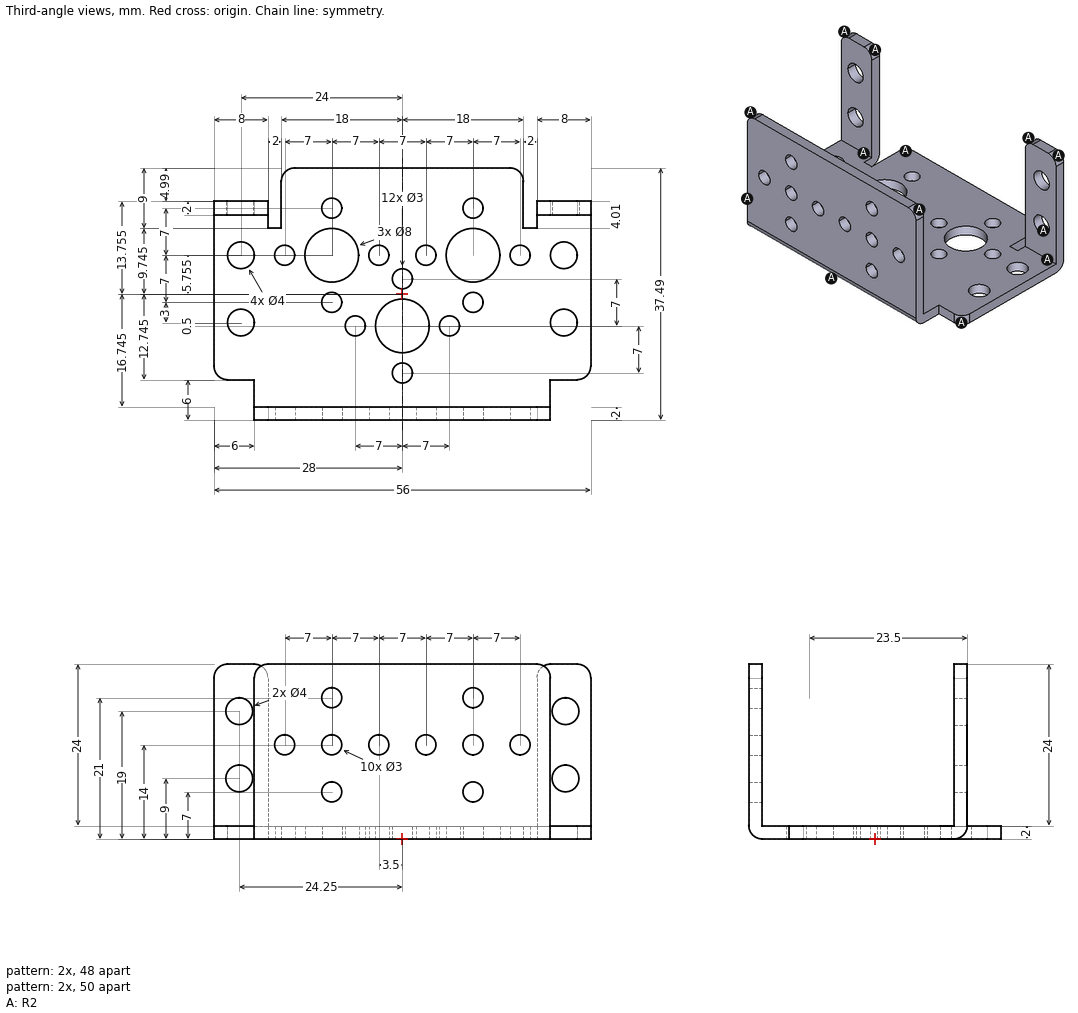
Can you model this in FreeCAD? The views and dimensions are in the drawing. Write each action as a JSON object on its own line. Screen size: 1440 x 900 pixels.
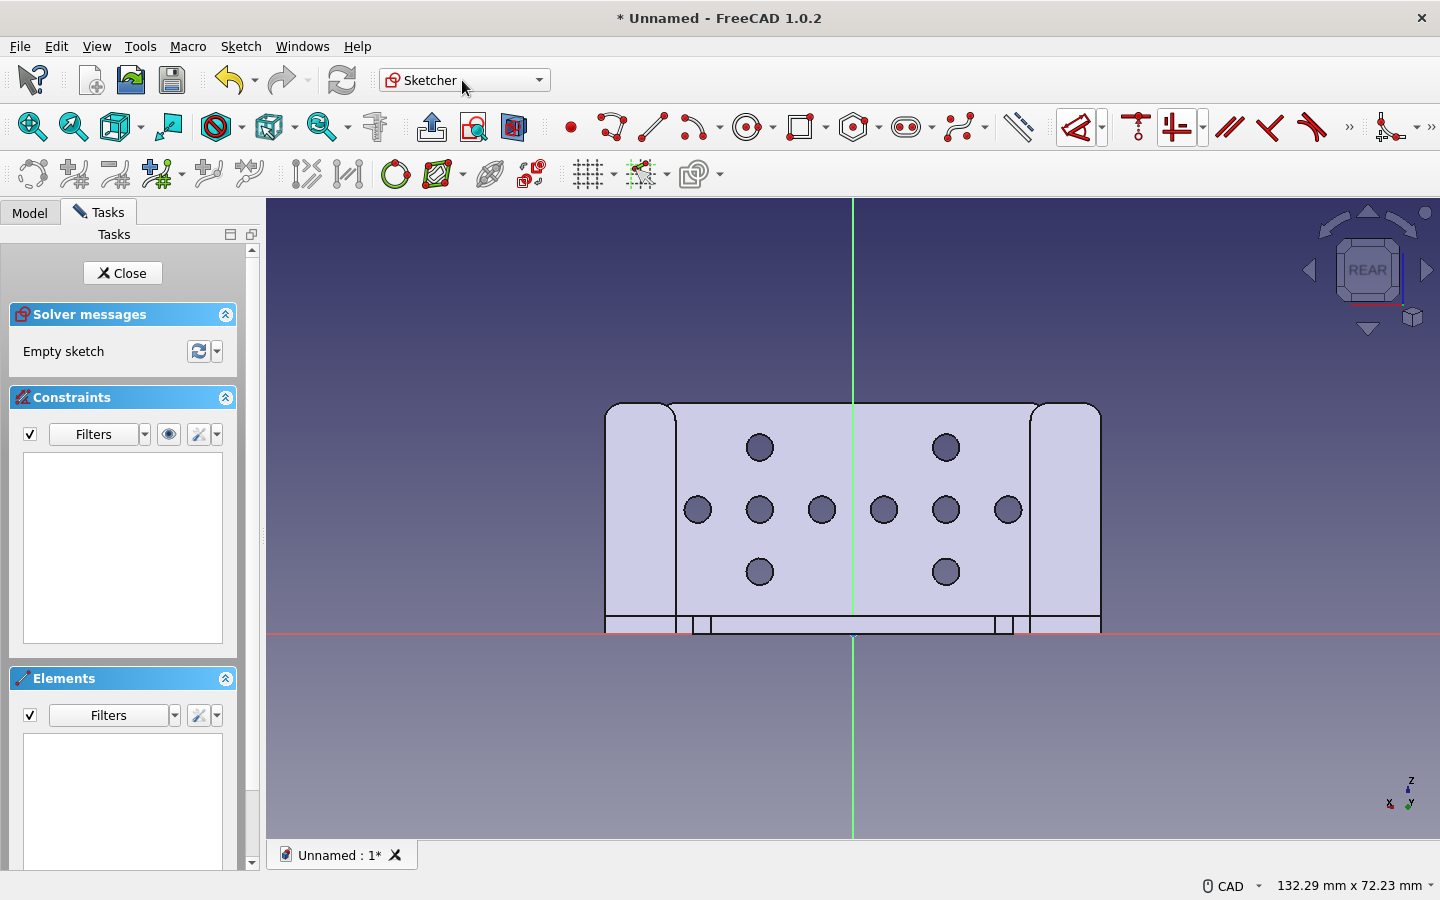
{"action": "key", "text": "q s"}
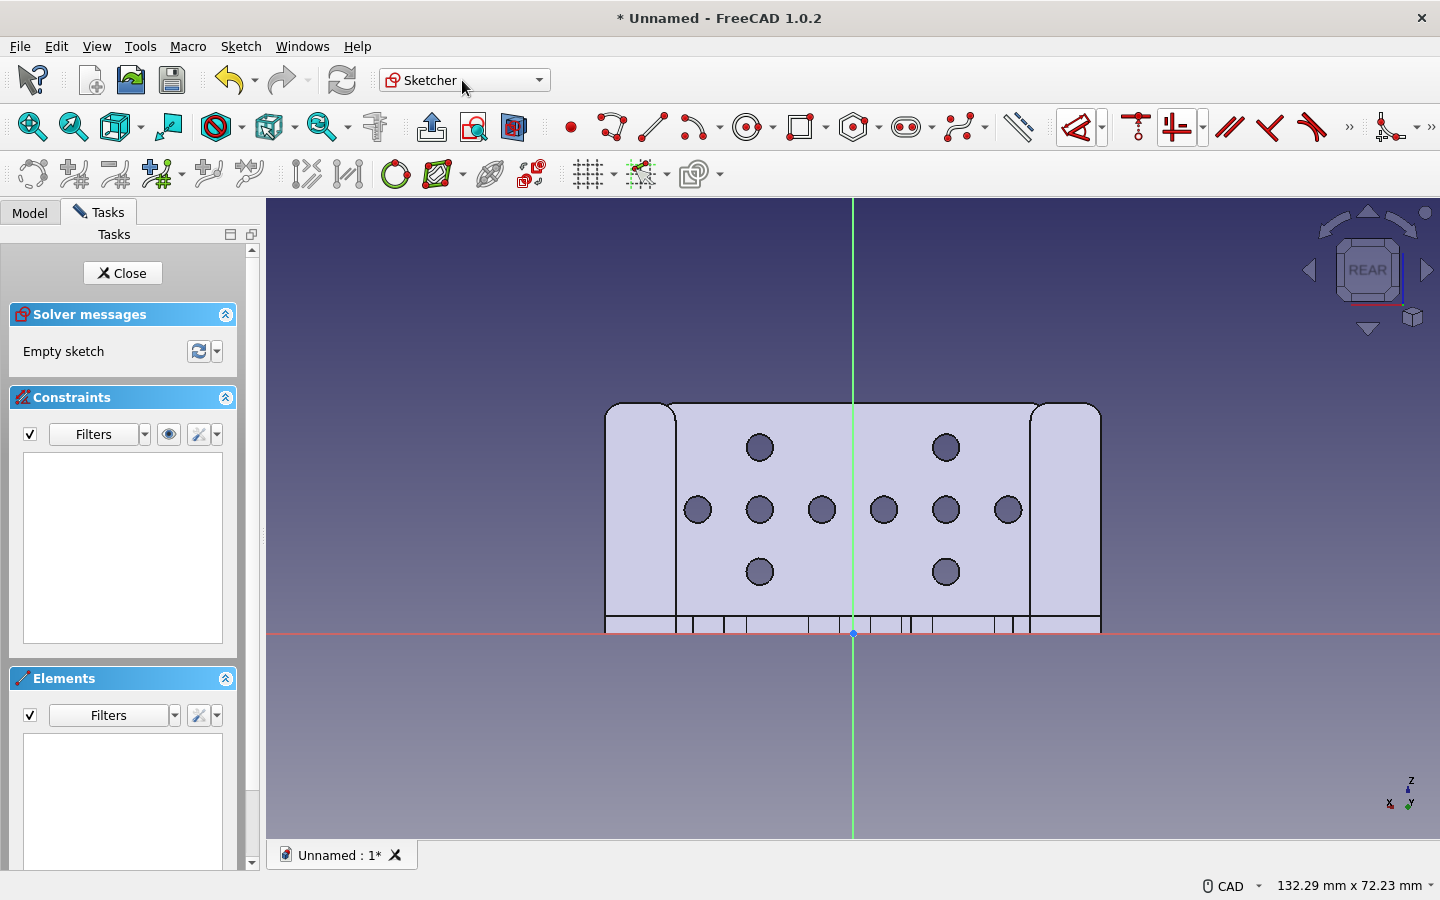
{"action": "scroll", "coordinate": [1120, 559], "scroll_direction": "up", "scroll_amount": 4}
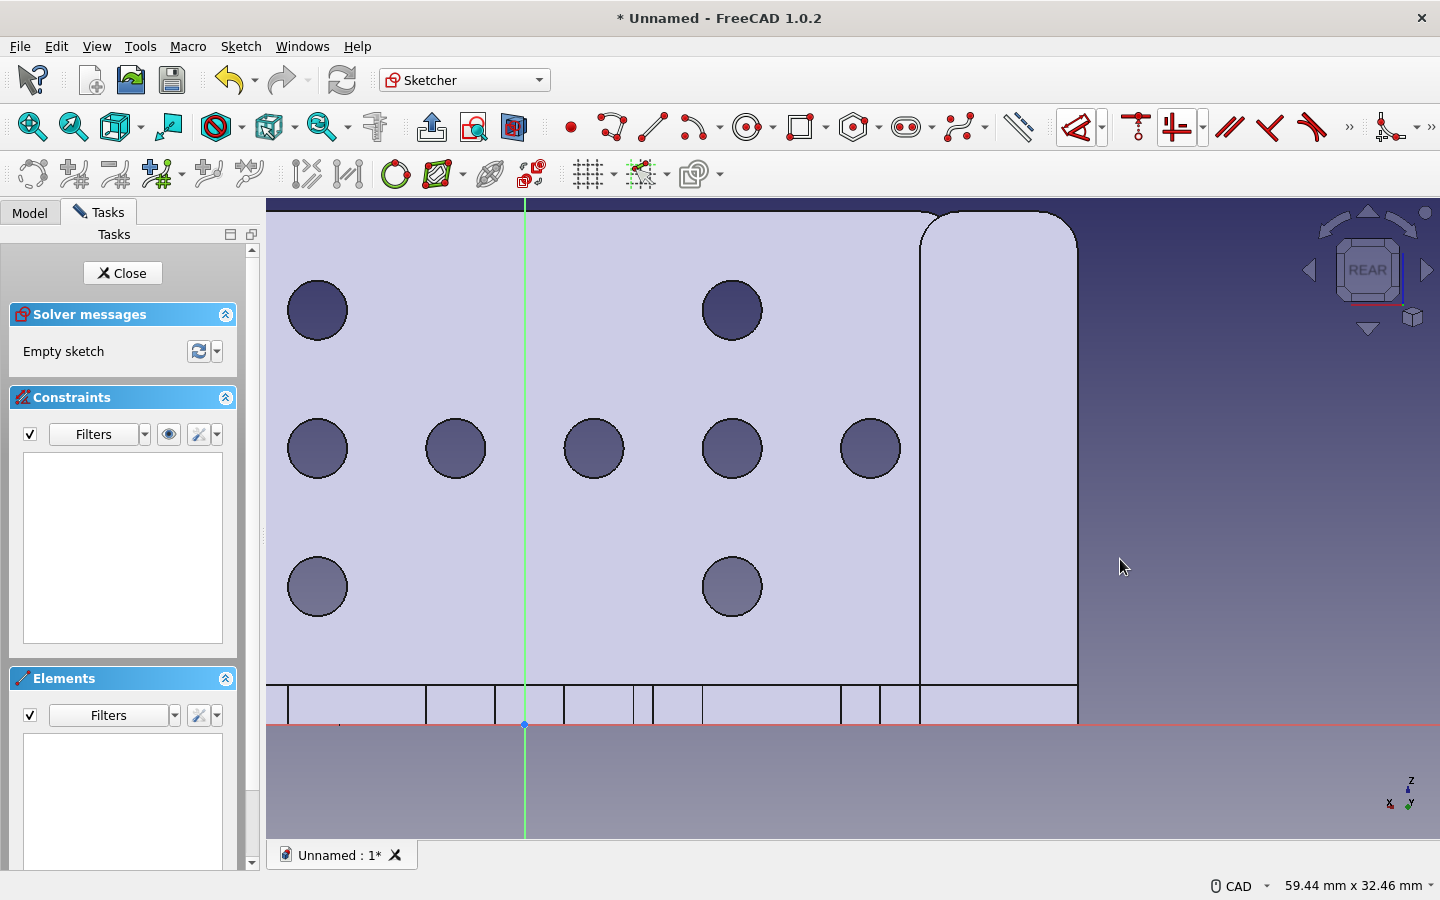
{"action": "left_click", "coordinate": [746, 128]}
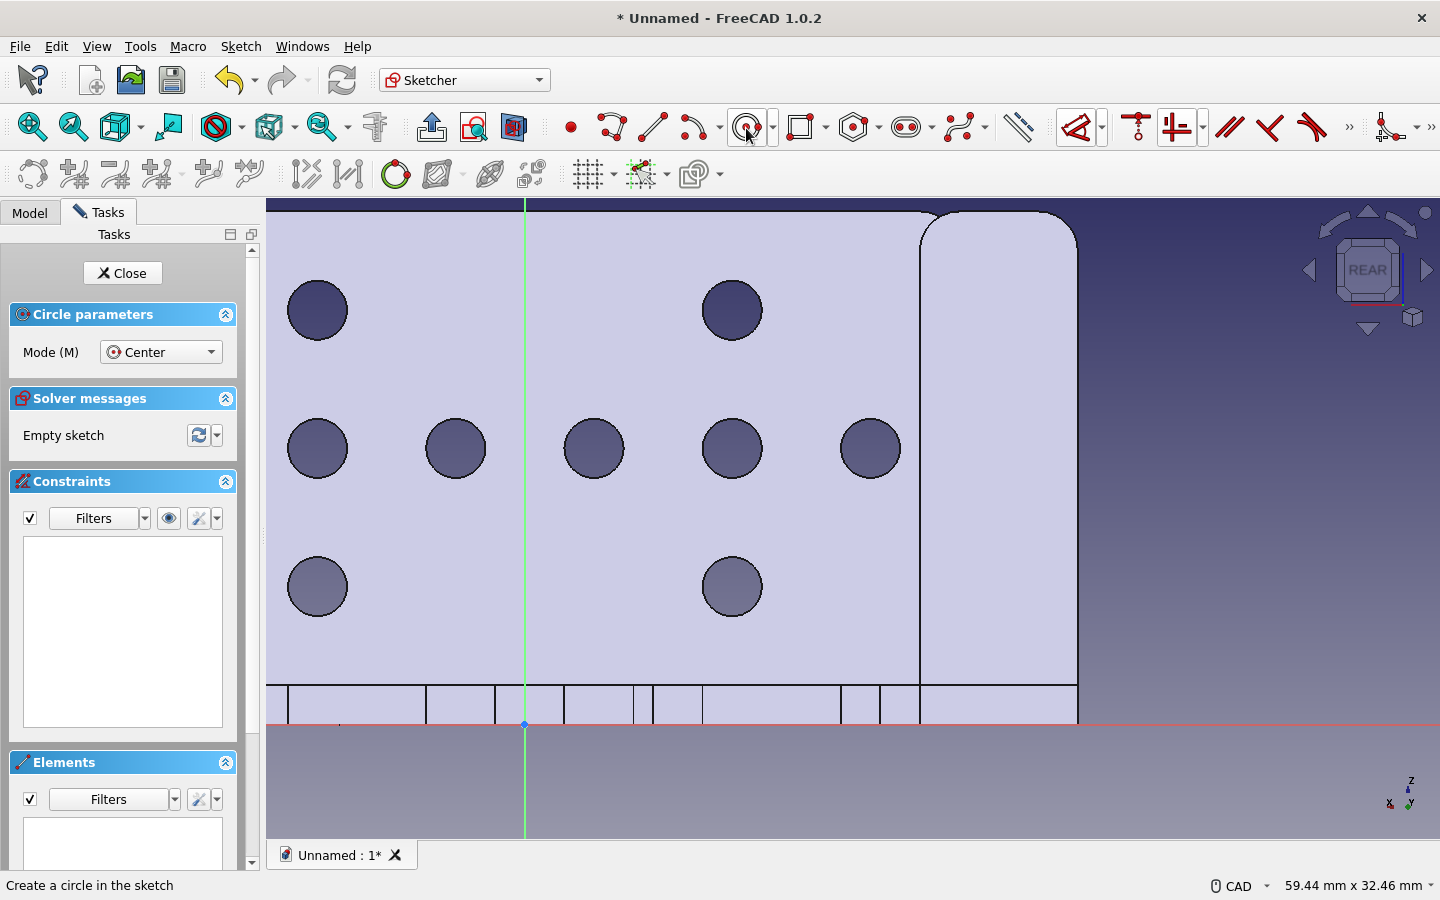
{"action": "left_click", "coordinate": [1004, 350]}
{"action": "mouse_move", "coordinate": [1032, 322]}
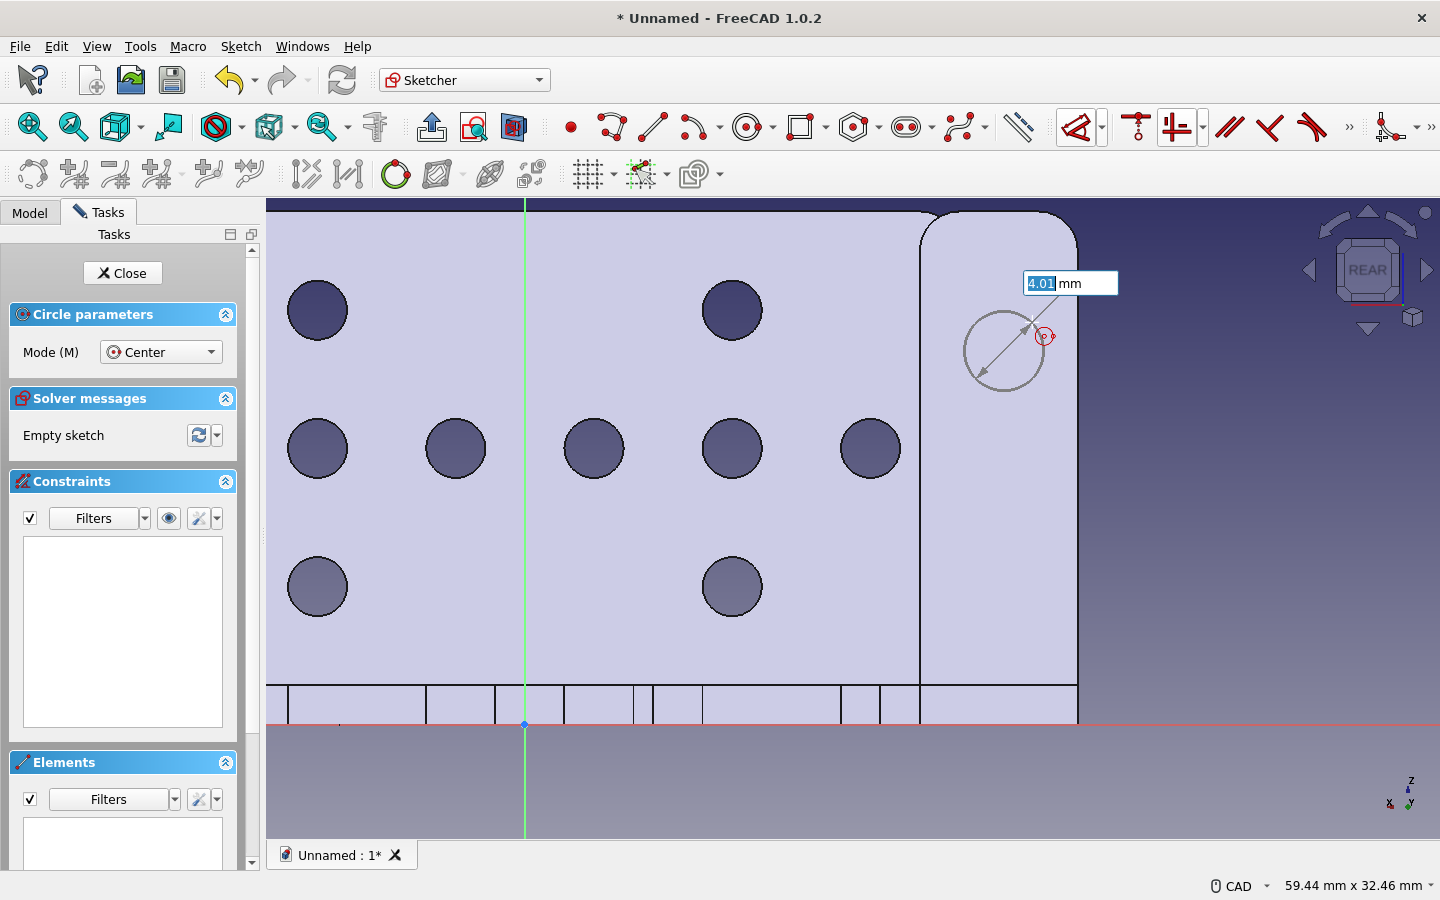
{"action": "type", "text": "4"}
{"action": "key", "text": "Return"}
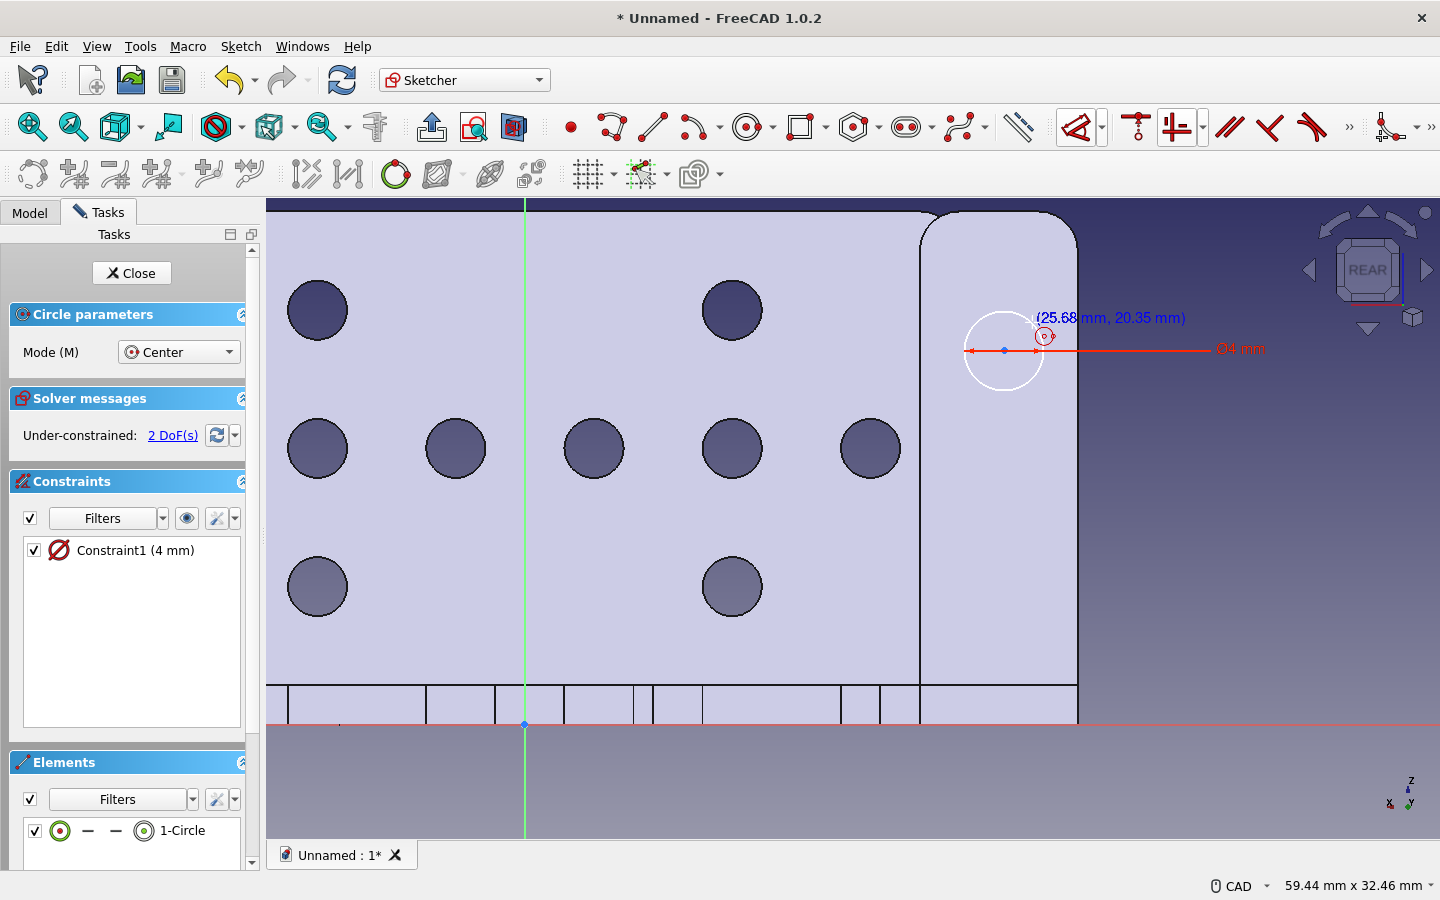
{"action": "left_click", "coordinate": [1004, 547]}
{"action": "mouse_move", "coordinate": [1032, 519]}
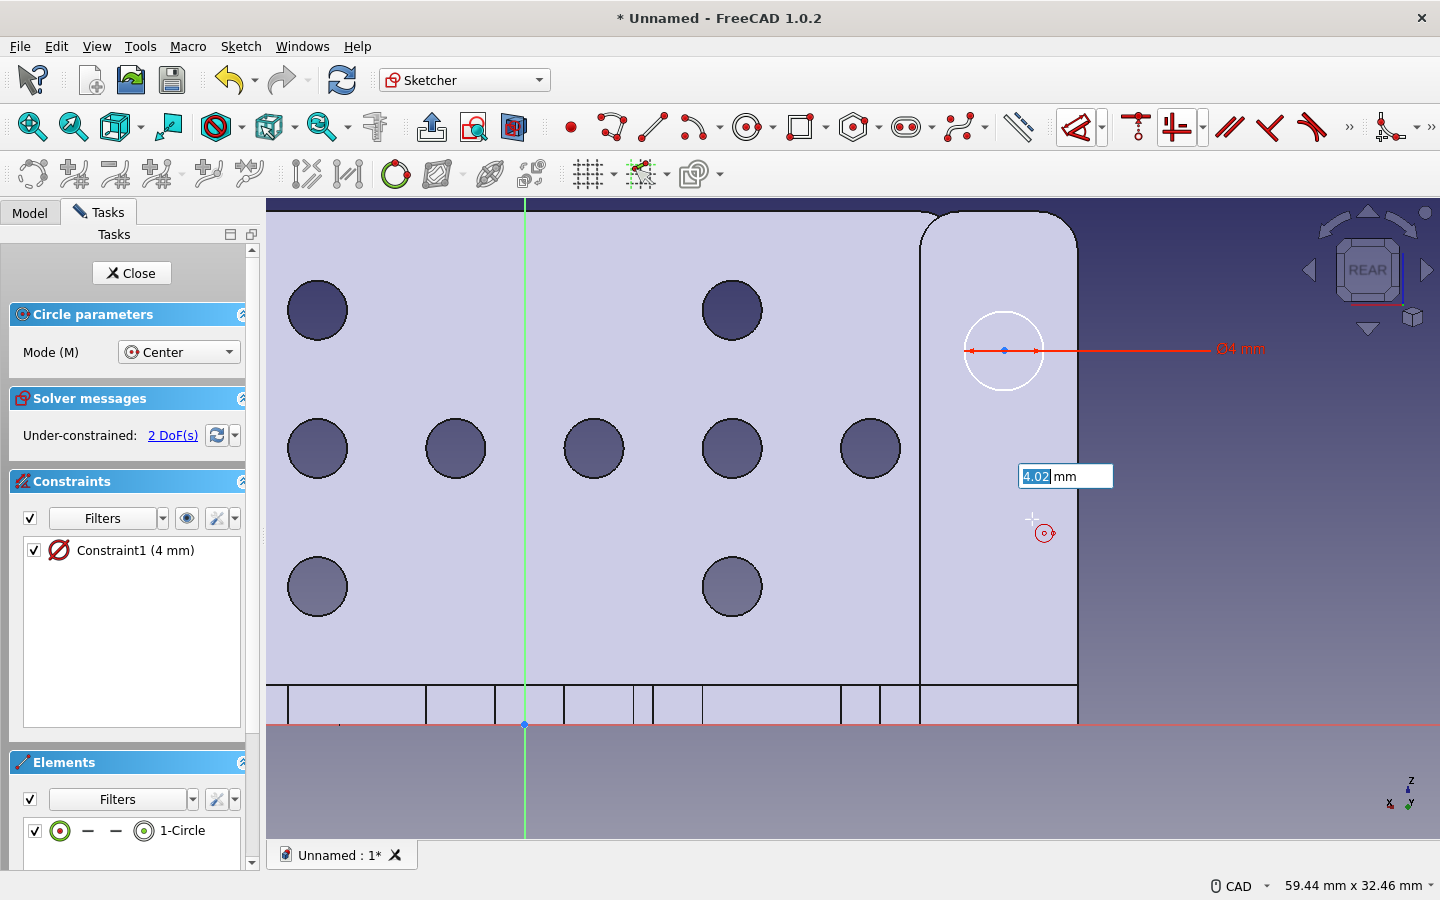
{"action": "type", "text": "4"}
{"action": "key", "text": "Return"}
{"action": "key", "text": "Escape"}